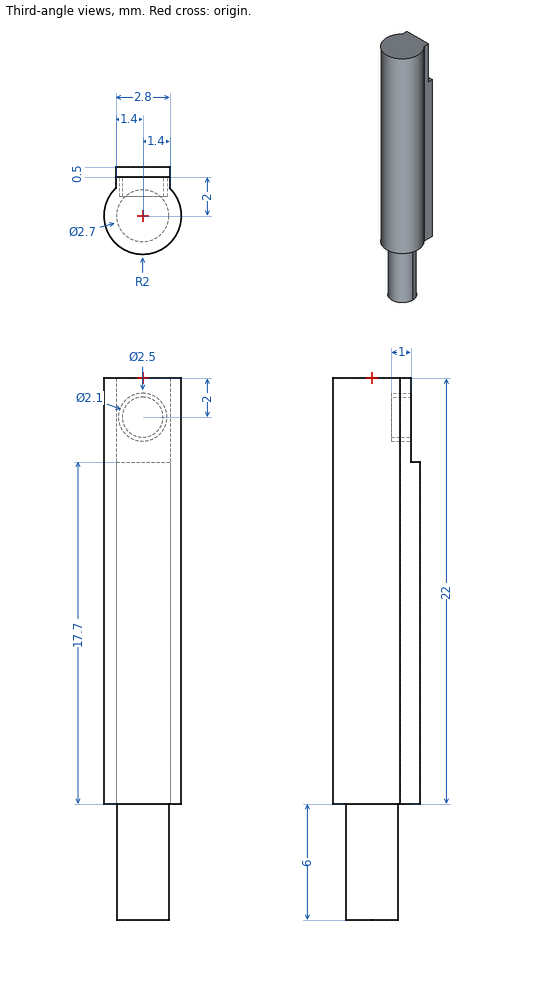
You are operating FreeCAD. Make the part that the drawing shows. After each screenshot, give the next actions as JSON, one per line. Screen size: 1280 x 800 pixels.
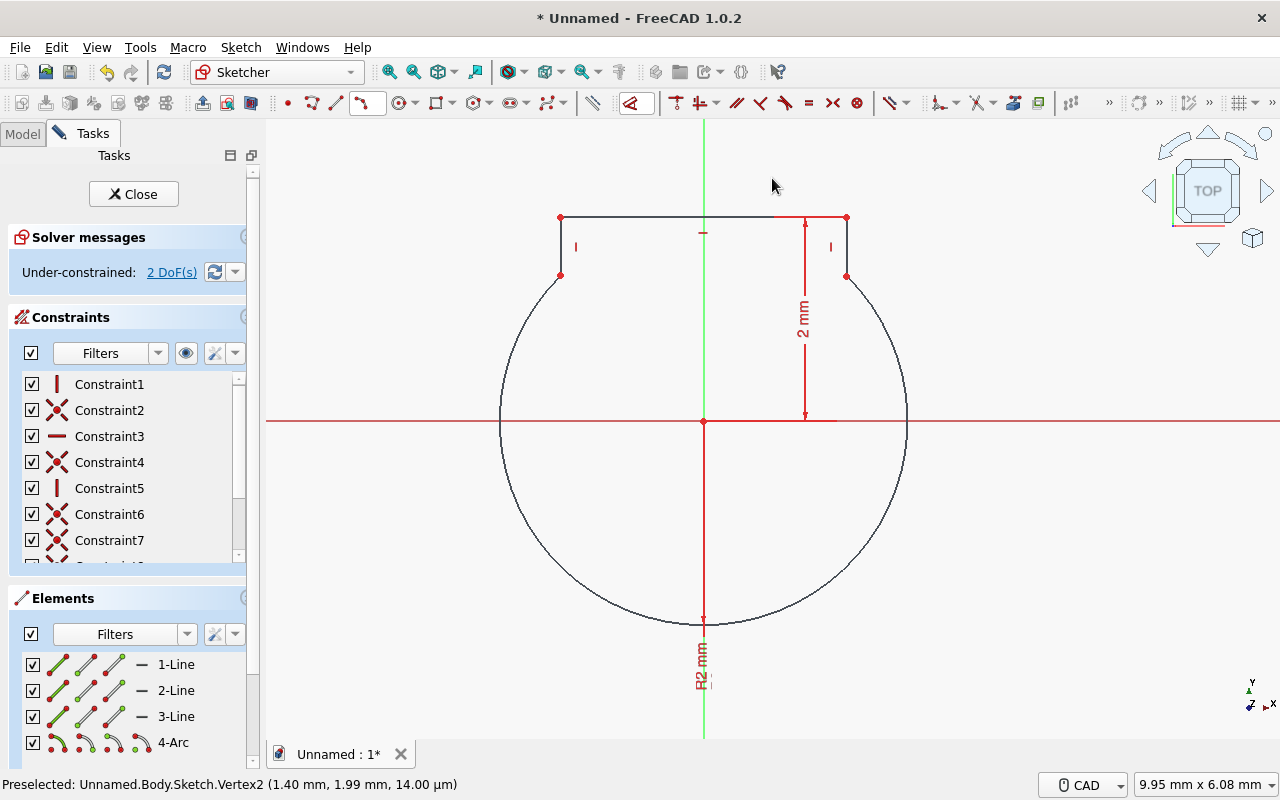
{"action": "left_click", "coordinate": [761, 217]}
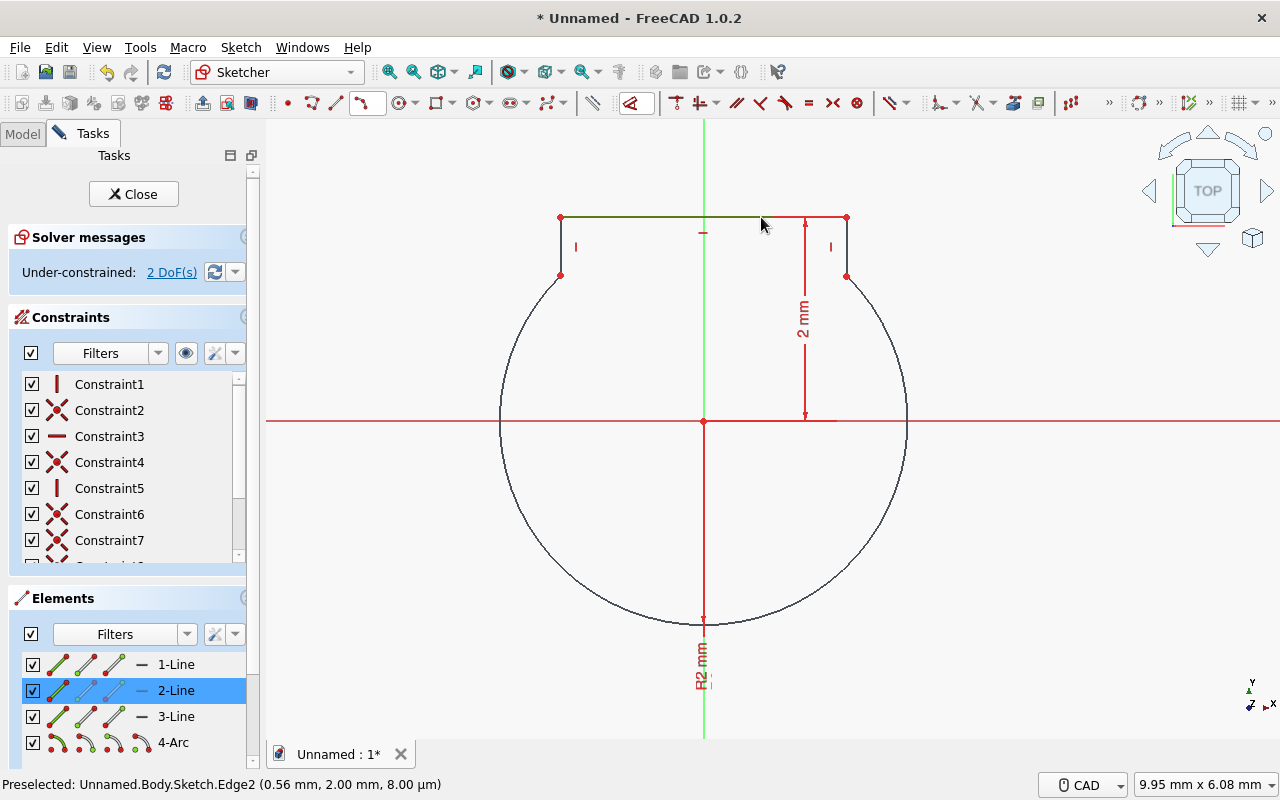
{"action": "left_click", "coordinate": [648, 104]}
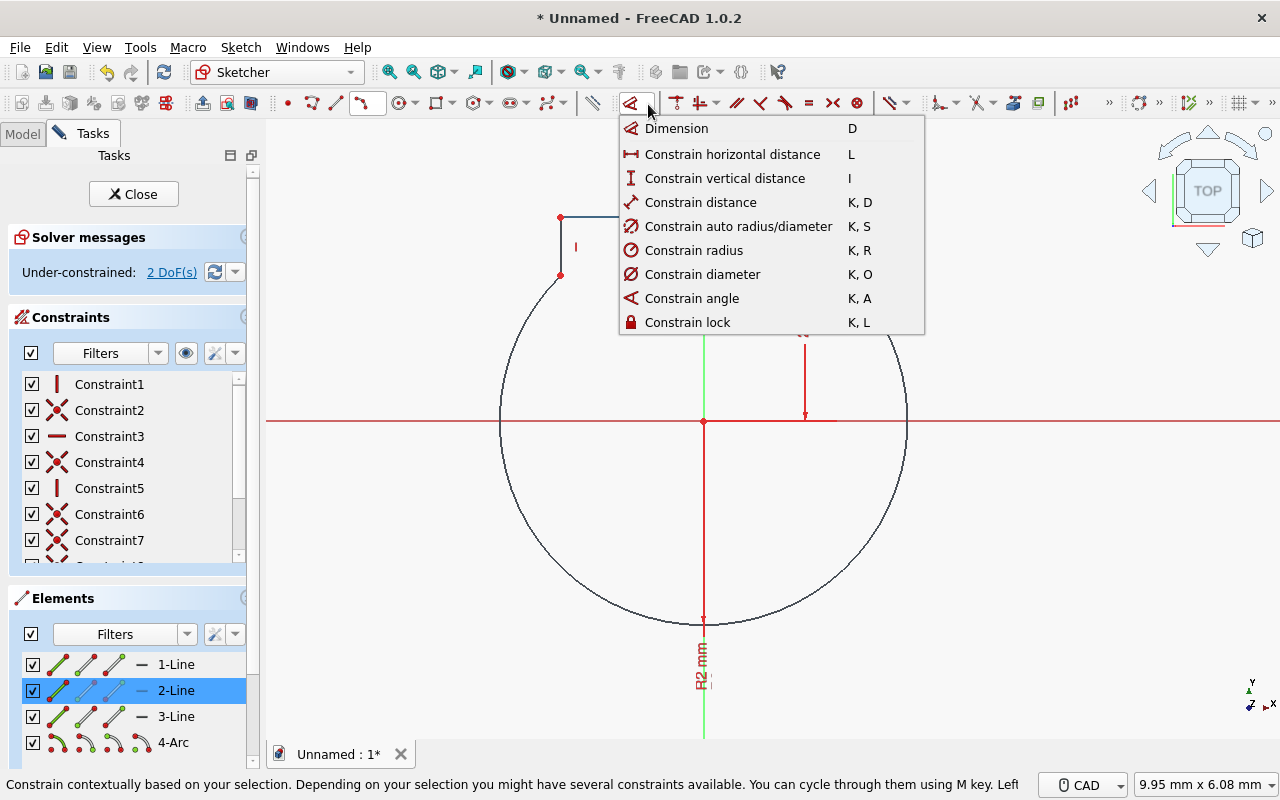
{"action": "left_click", "coordinate": [772, 154]}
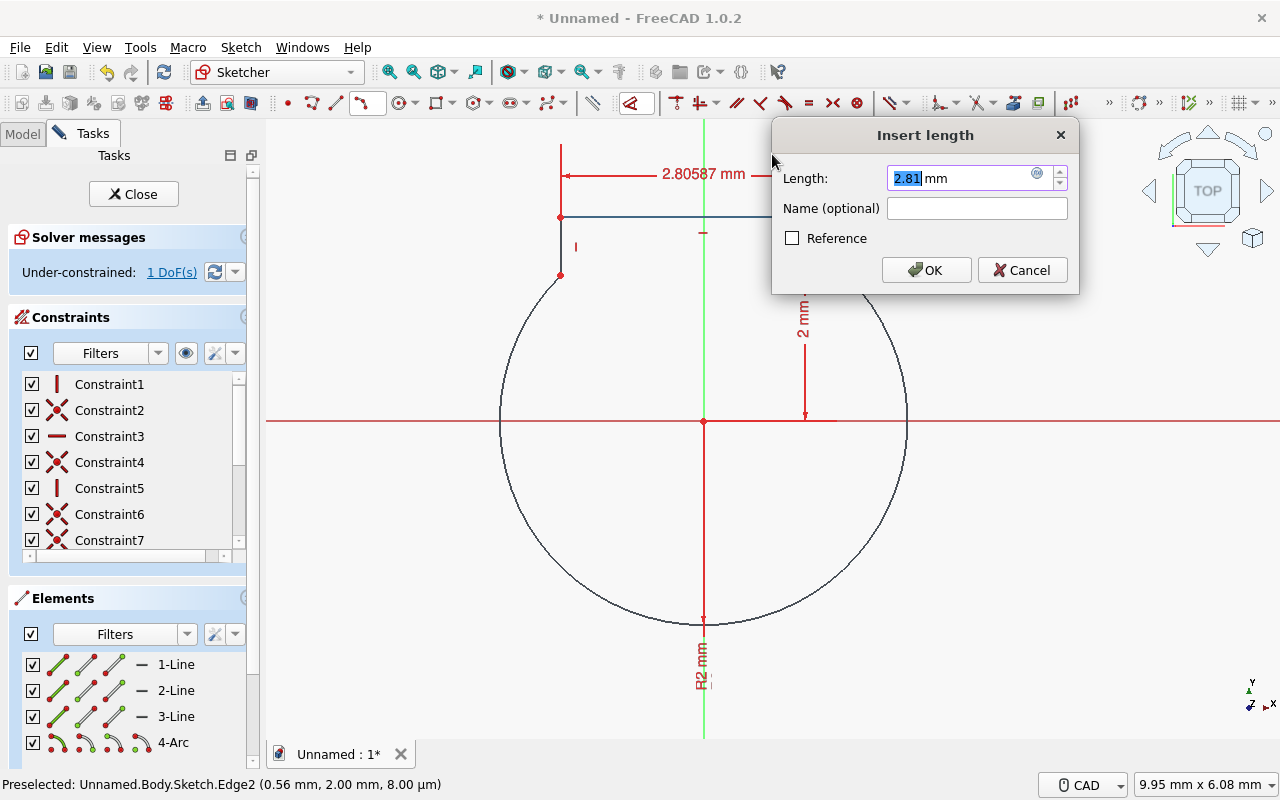
{"action": "type", "text": "2.8"}
{"action": "key", "text": "Return"}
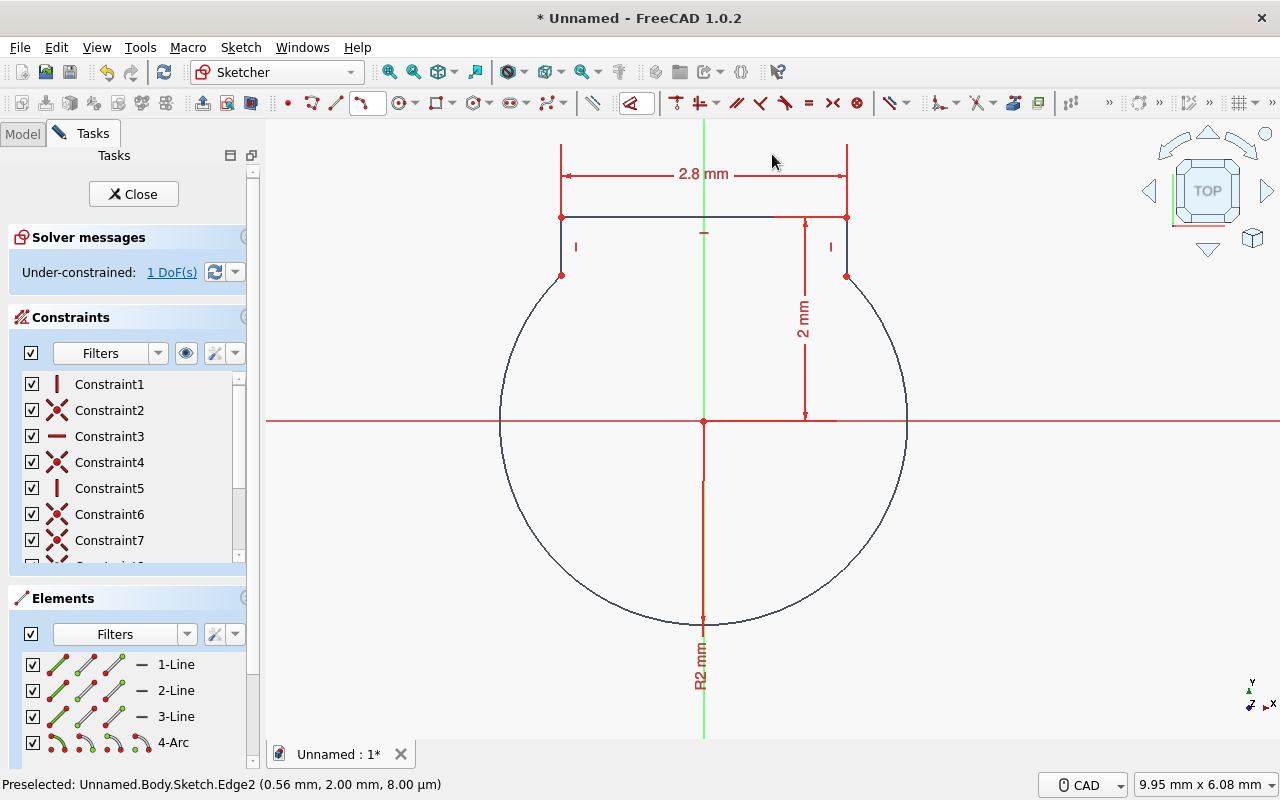
{"action": "left_click", "coordinate": [847, 276]}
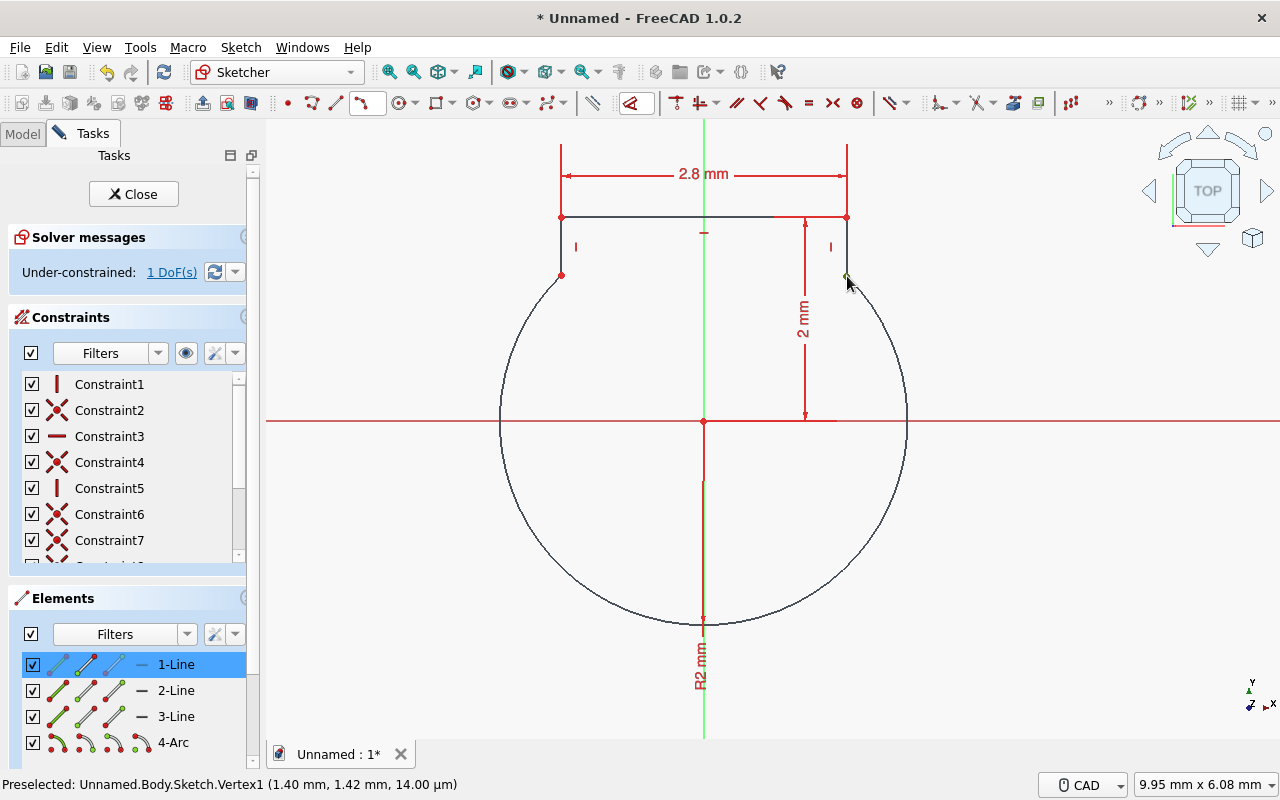
{"action": "key", "text": "l"}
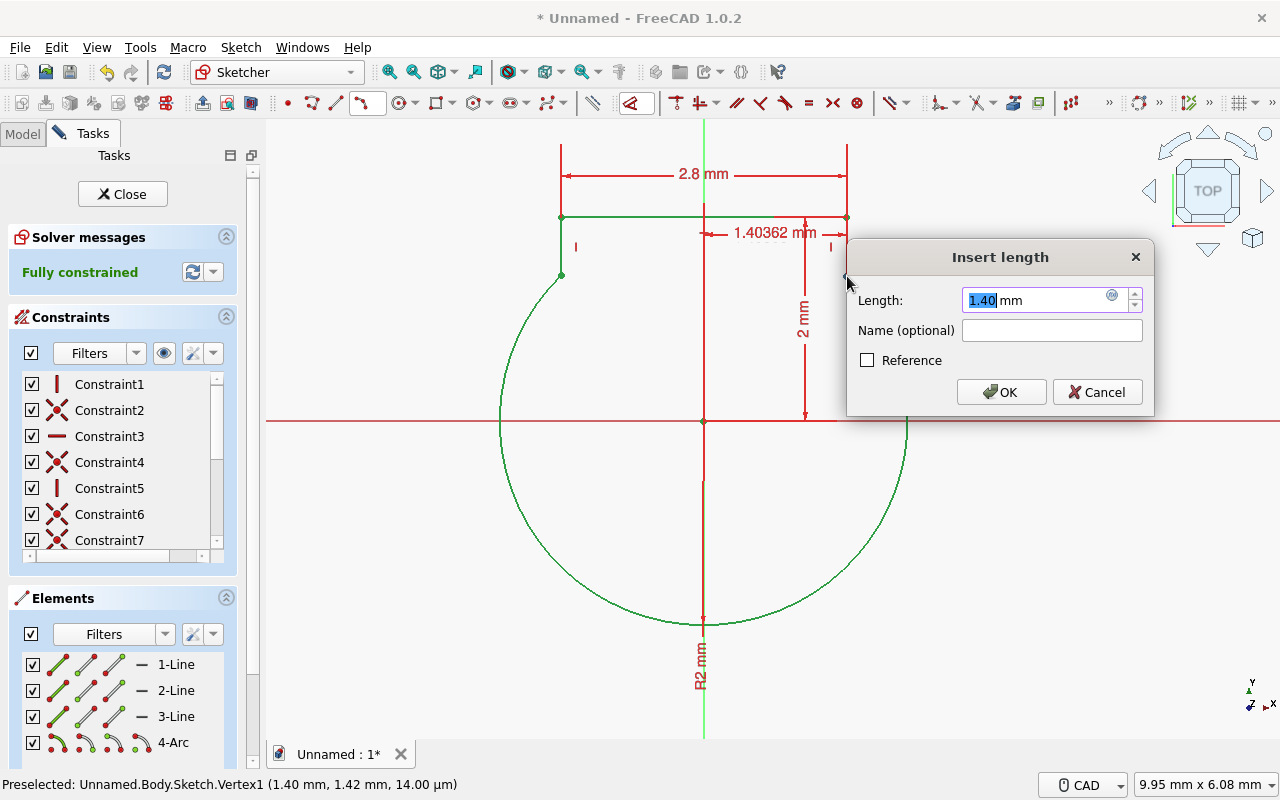
{"action": "type", "text": "1.4"}
{"action": "key", "text": "Return"}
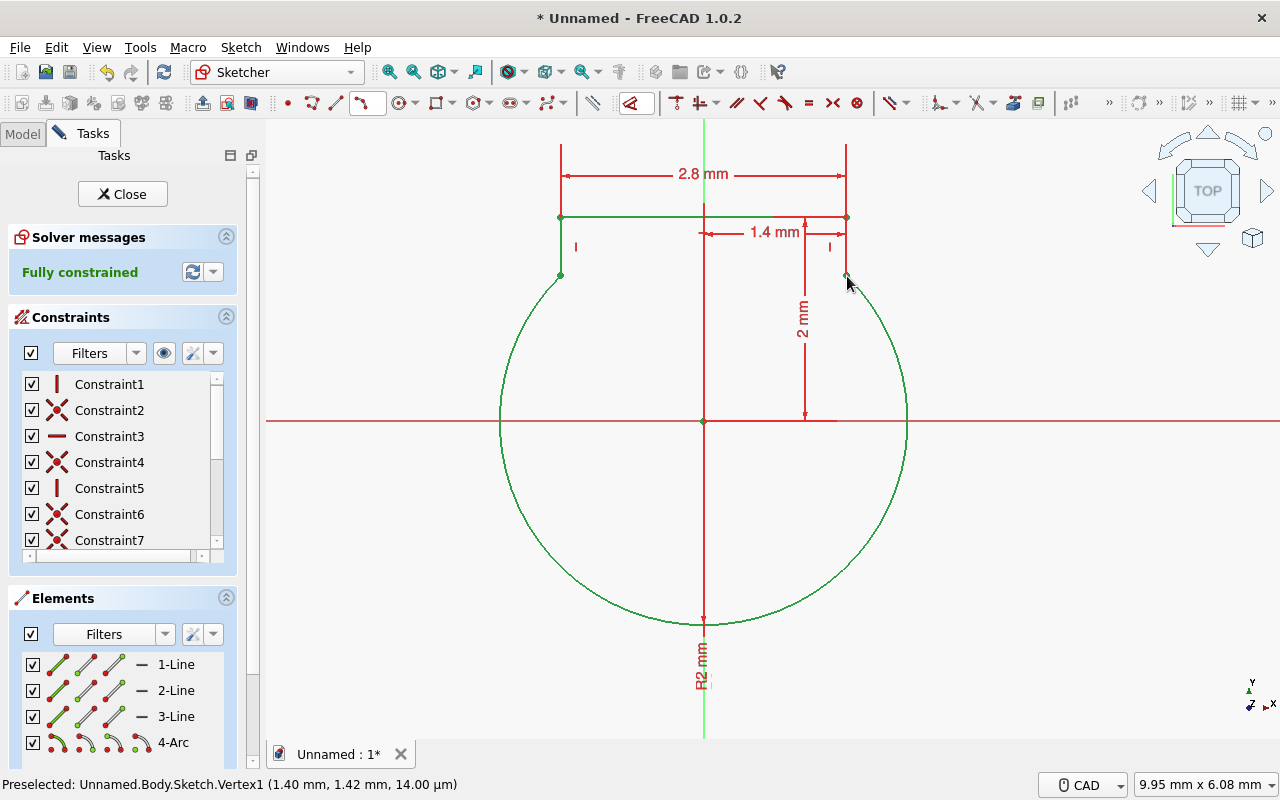
{"action": "left_click", "coordinate": [123, 194]}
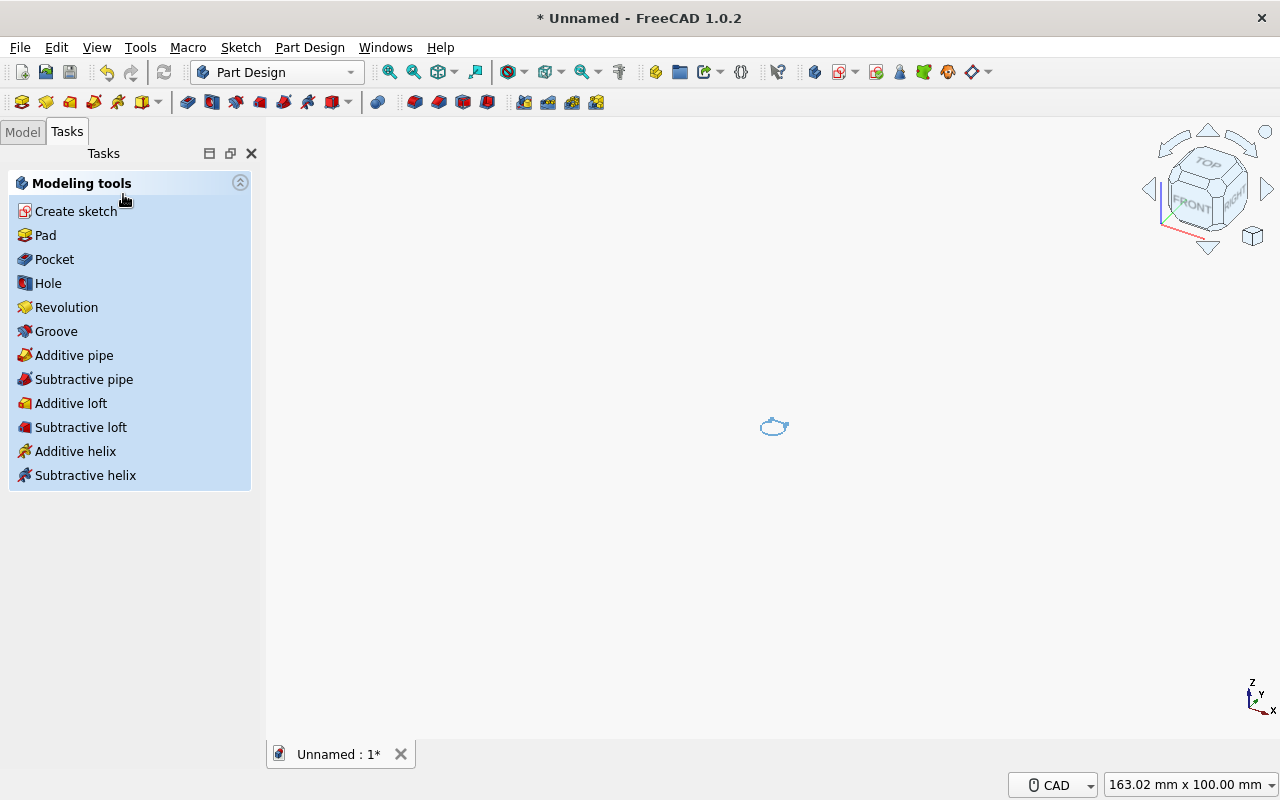
{"action": "left_click", "coordinate": [22, 102]}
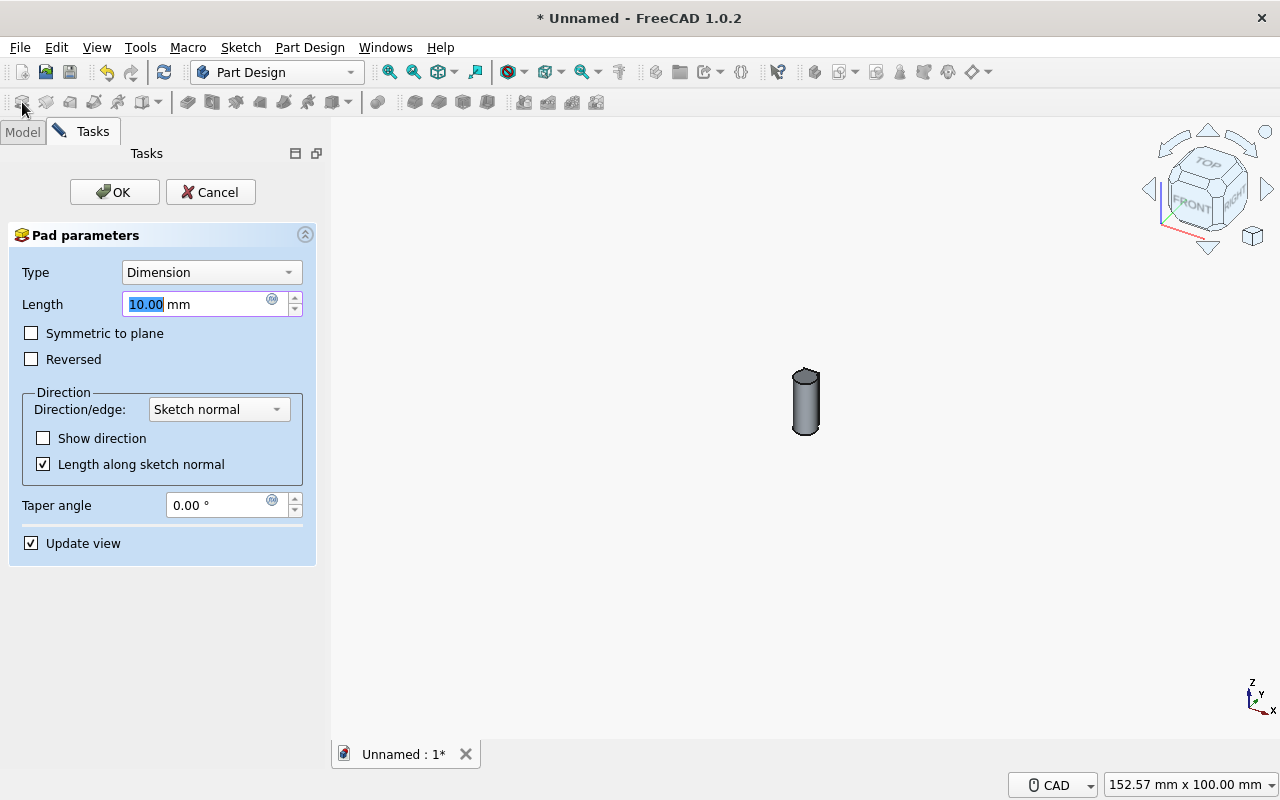
{"action": "type", "text": "22"}
{"action": "key", "text": "Tab"}